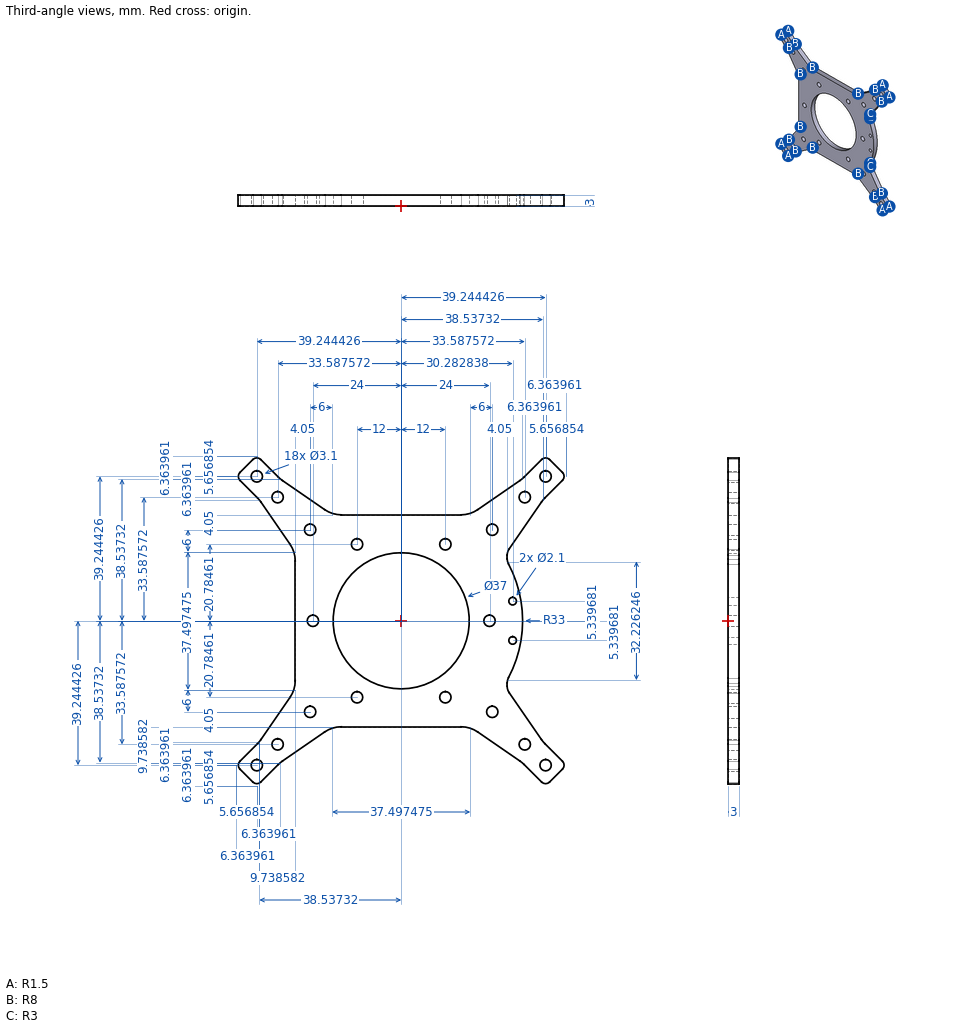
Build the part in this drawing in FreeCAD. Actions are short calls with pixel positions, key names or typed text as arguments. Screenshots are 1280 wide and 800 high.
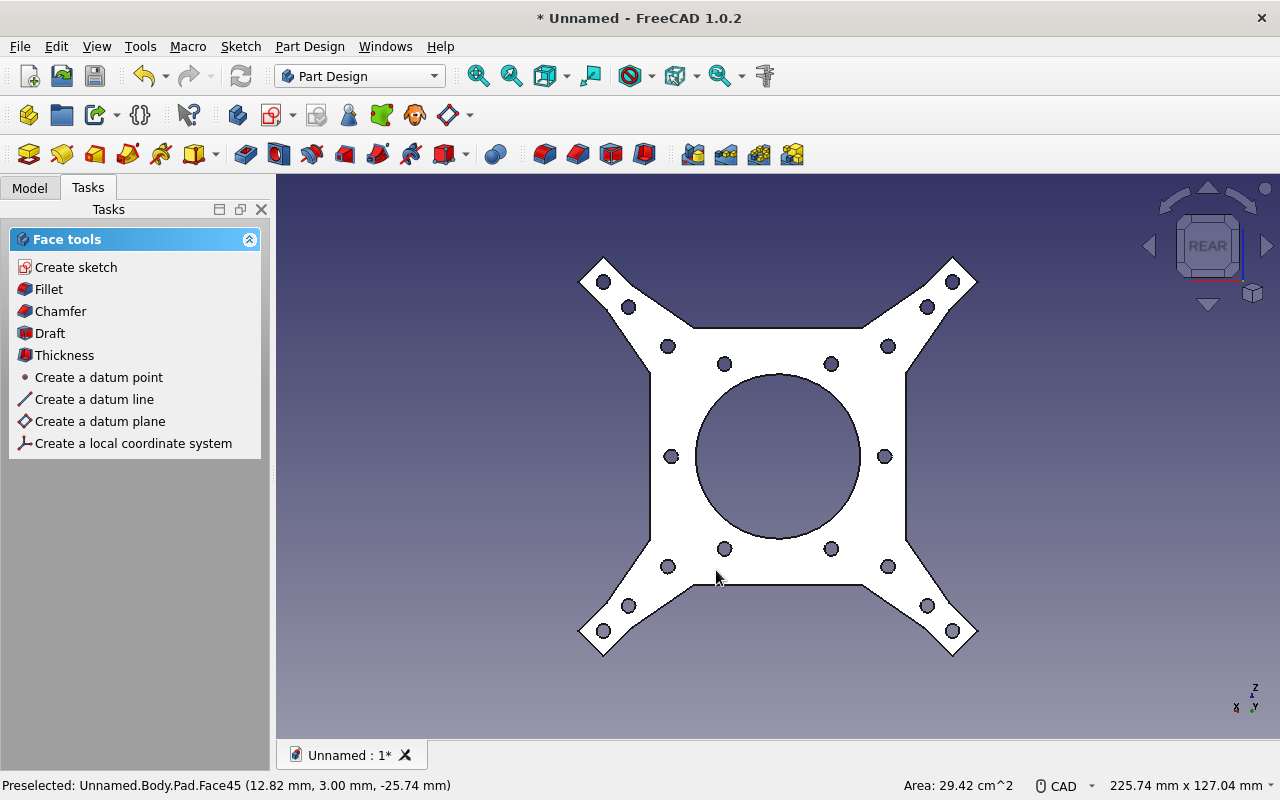
click(270, 116)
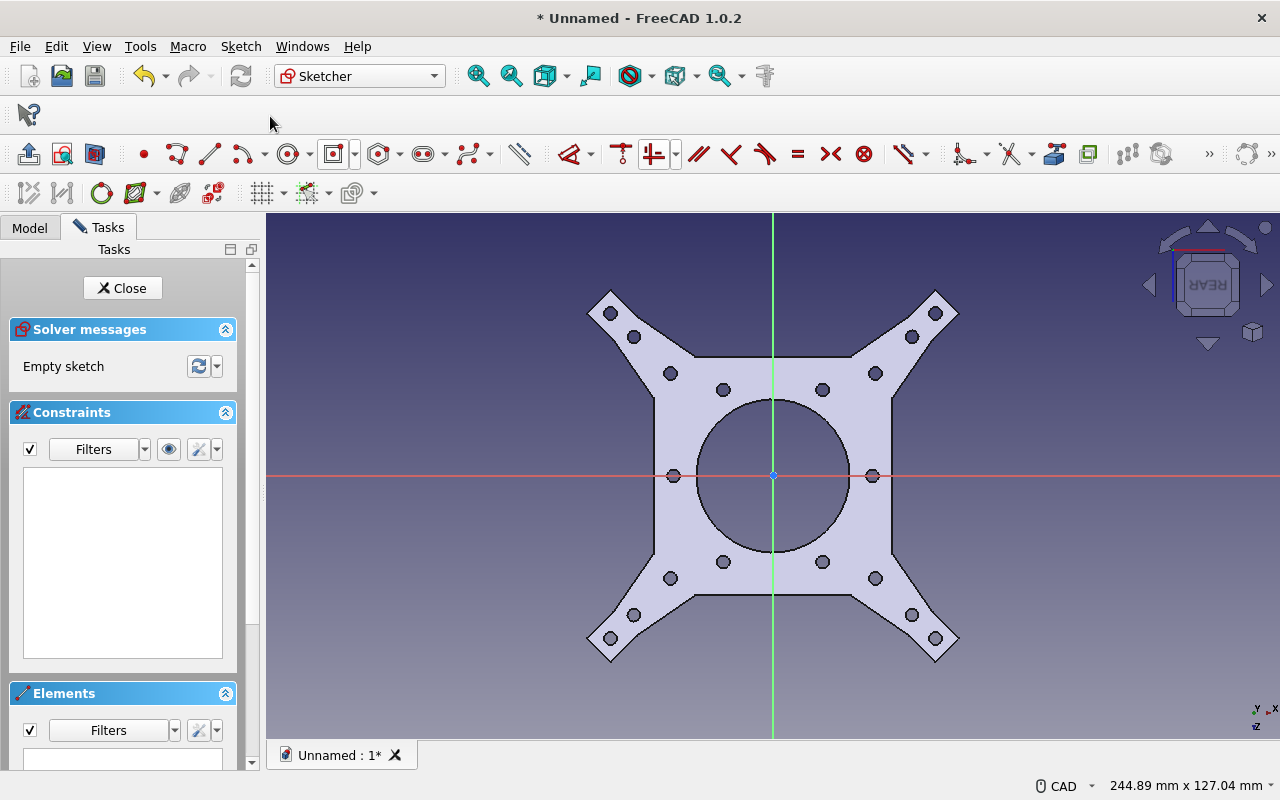
scroll(921, 476, up, 5)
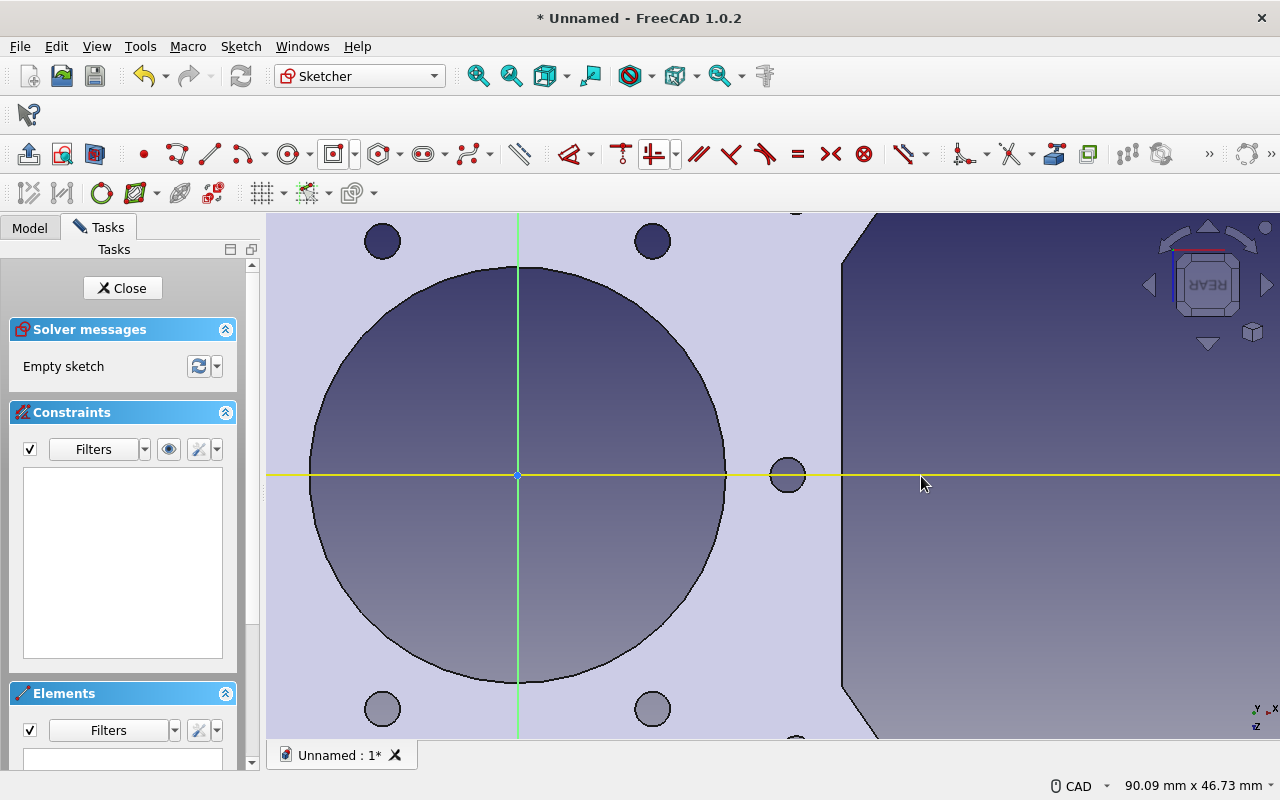
click(210, 154)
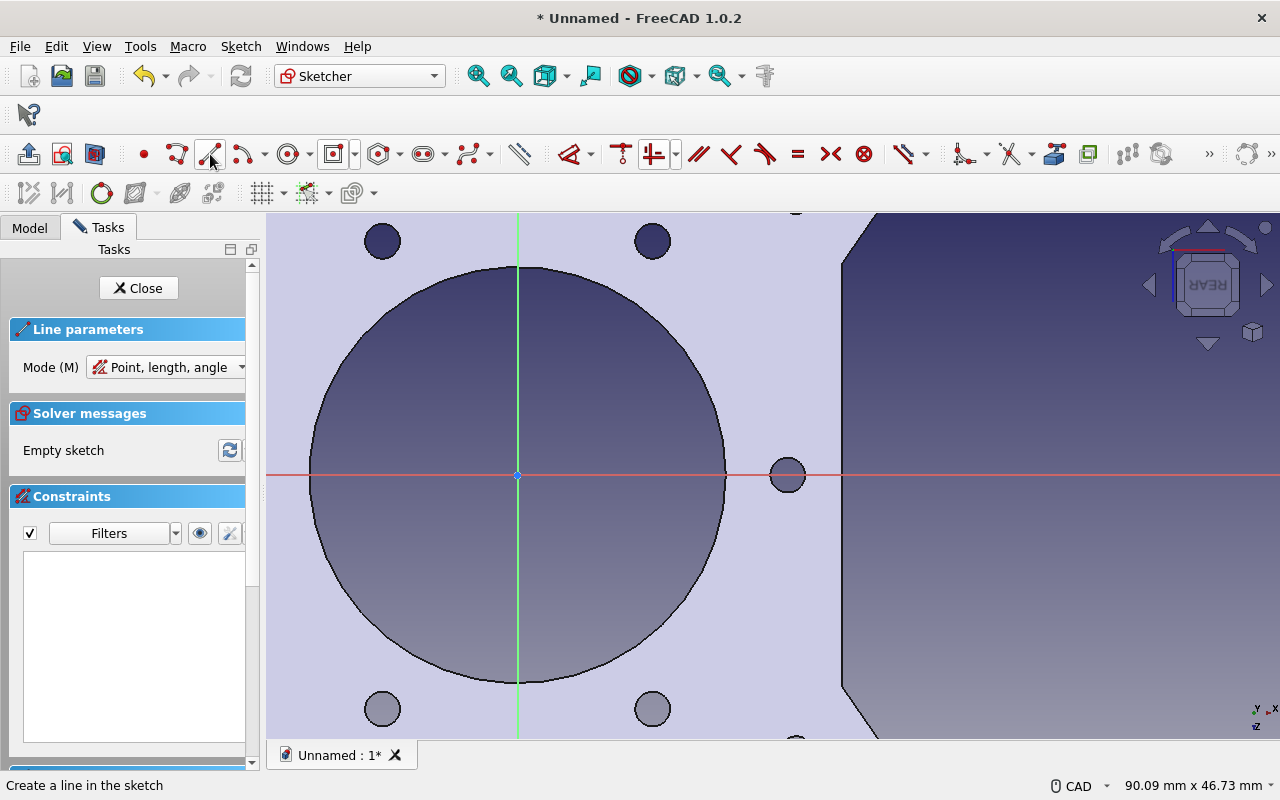
click(842, 294)
click(842, 656)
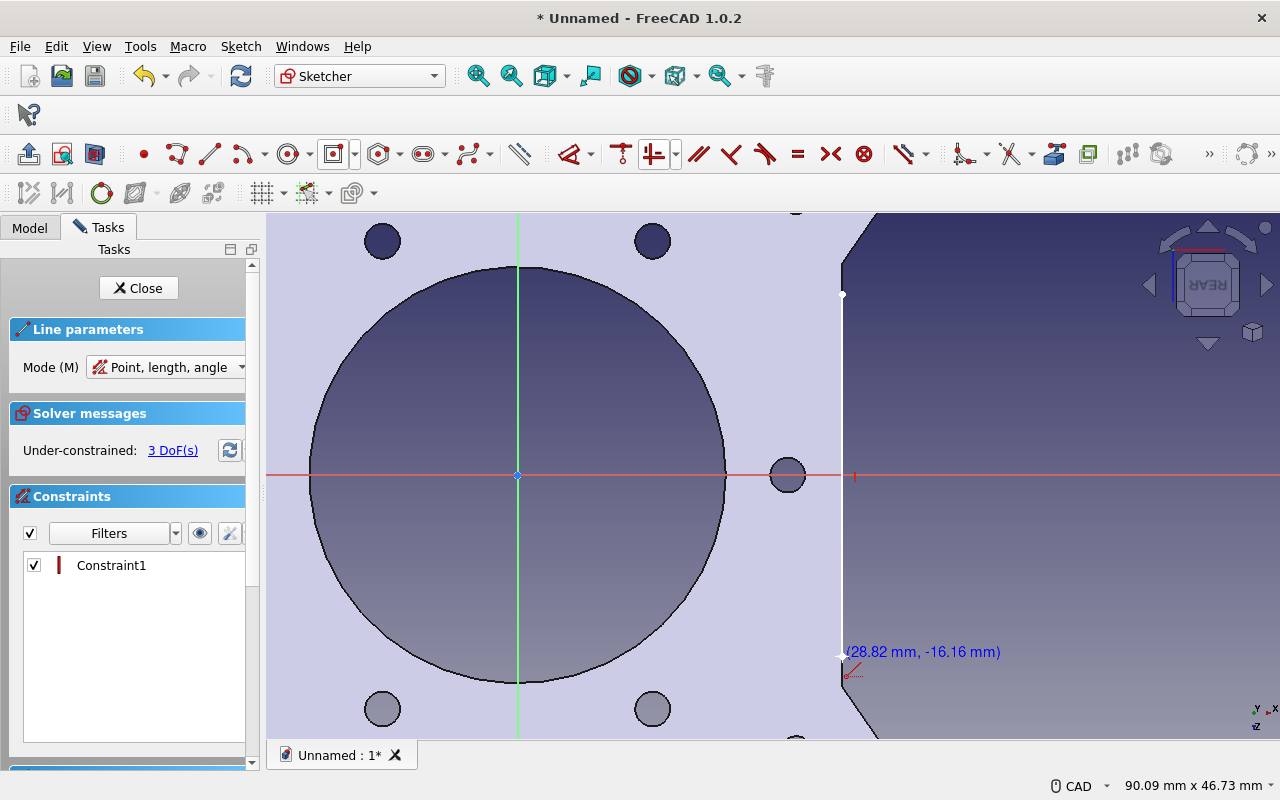
key(g)
key(3)
key(a)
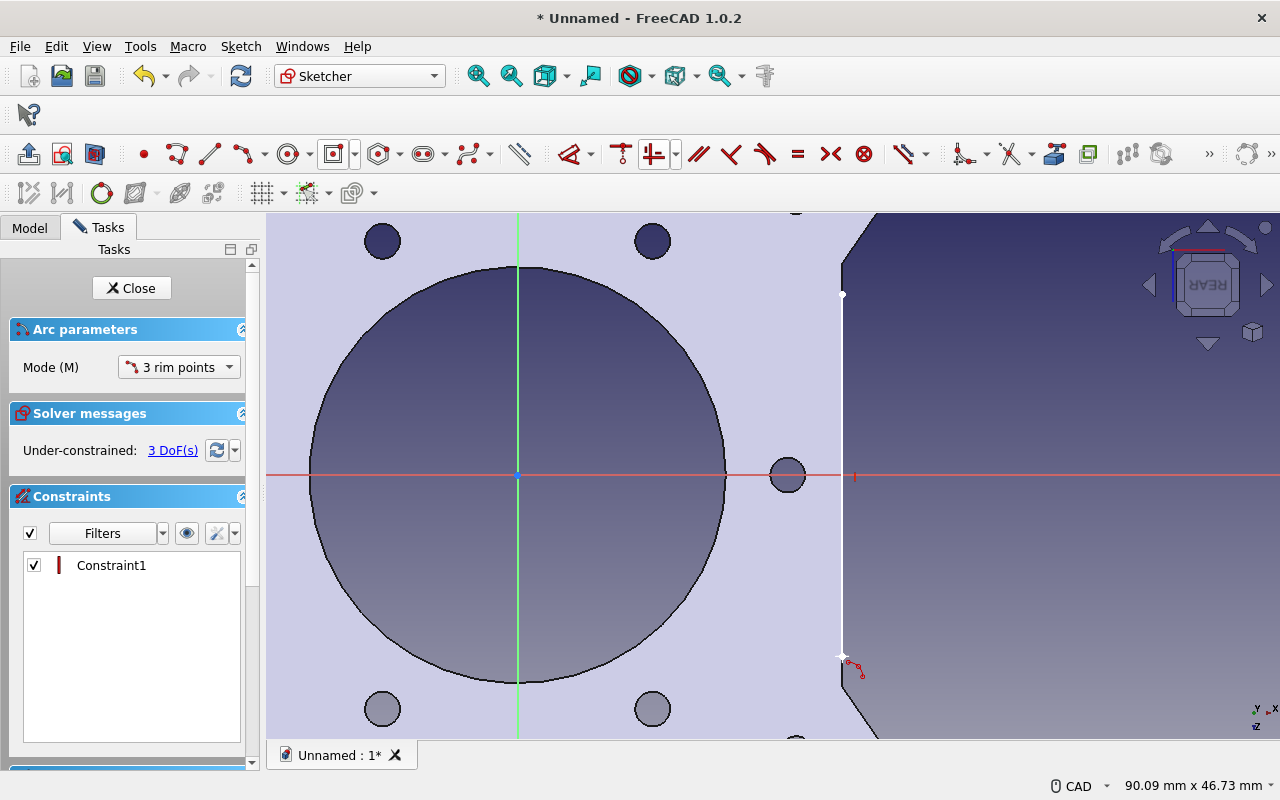
click(842, 657)
click(842, 295)
click(887, 513)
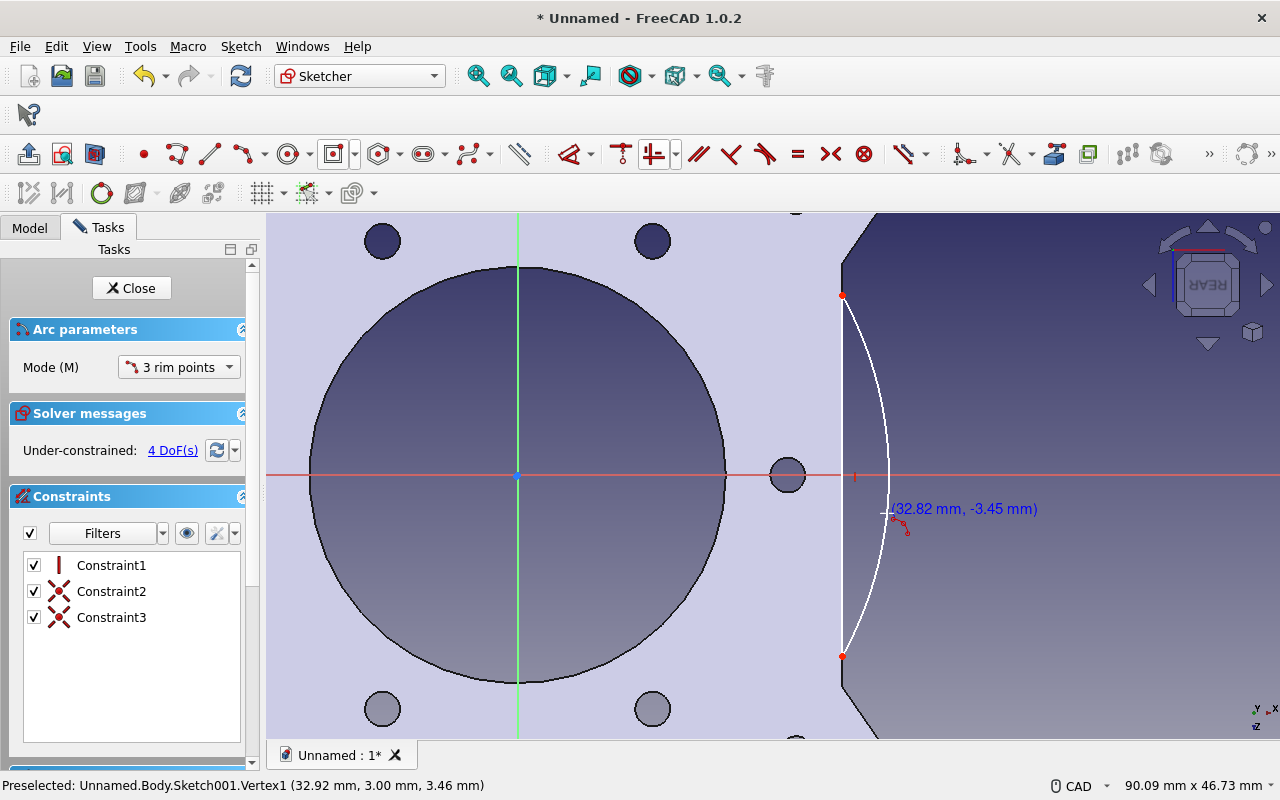
click(288, 154)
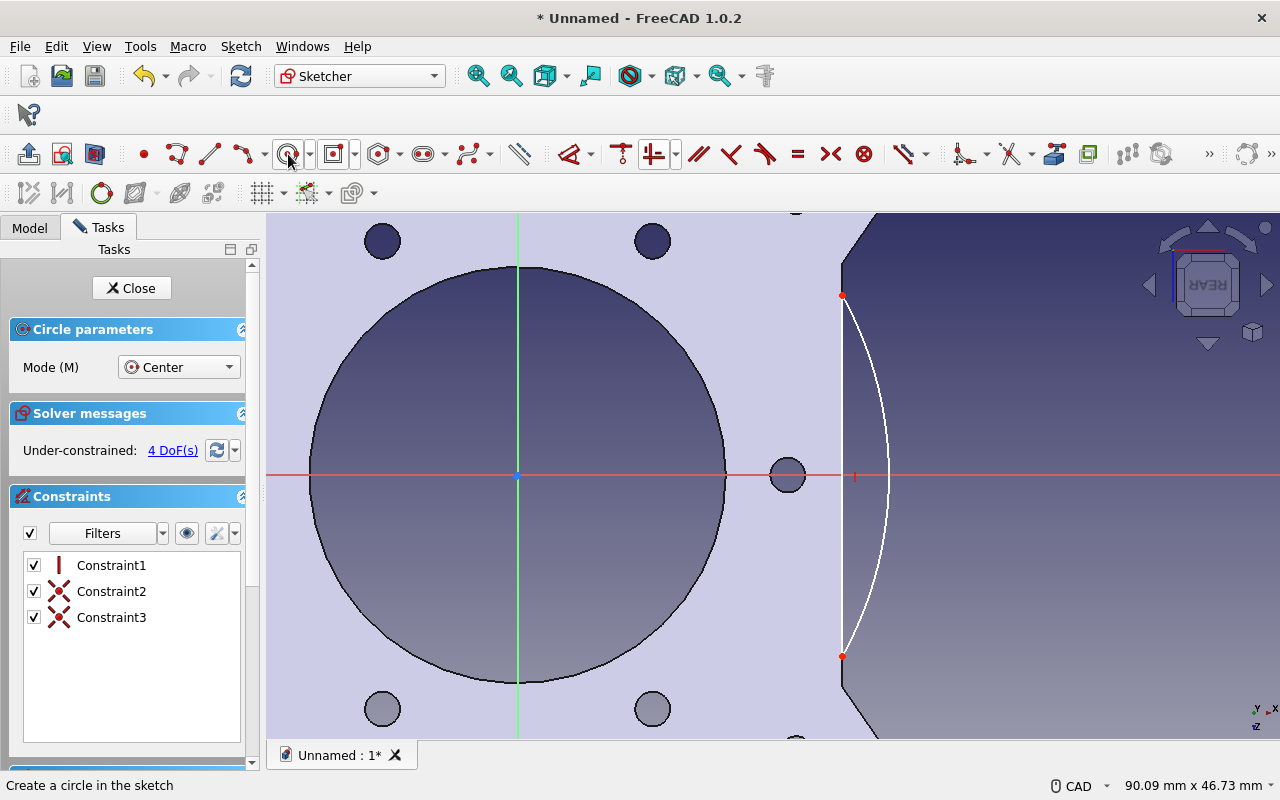
scroll(858, 535, up, 4)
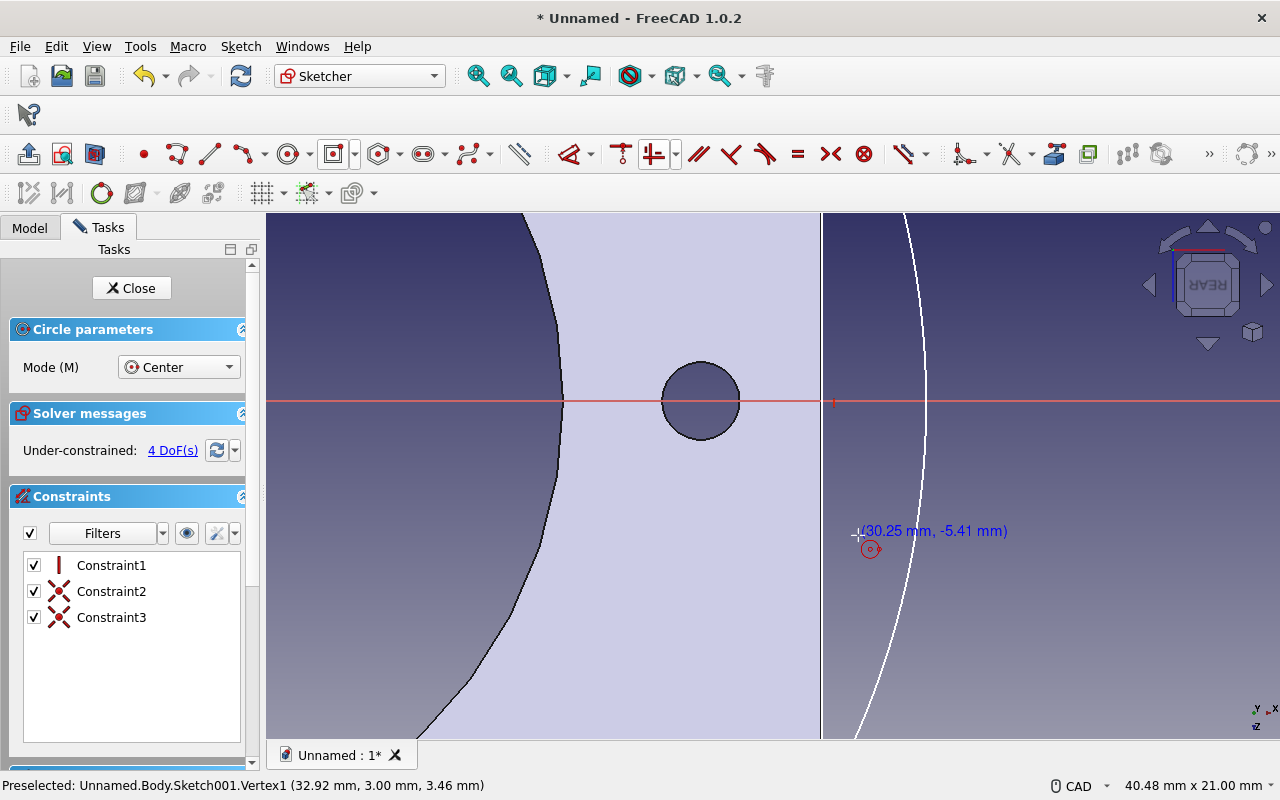
click(858, 535)
click(877, 516)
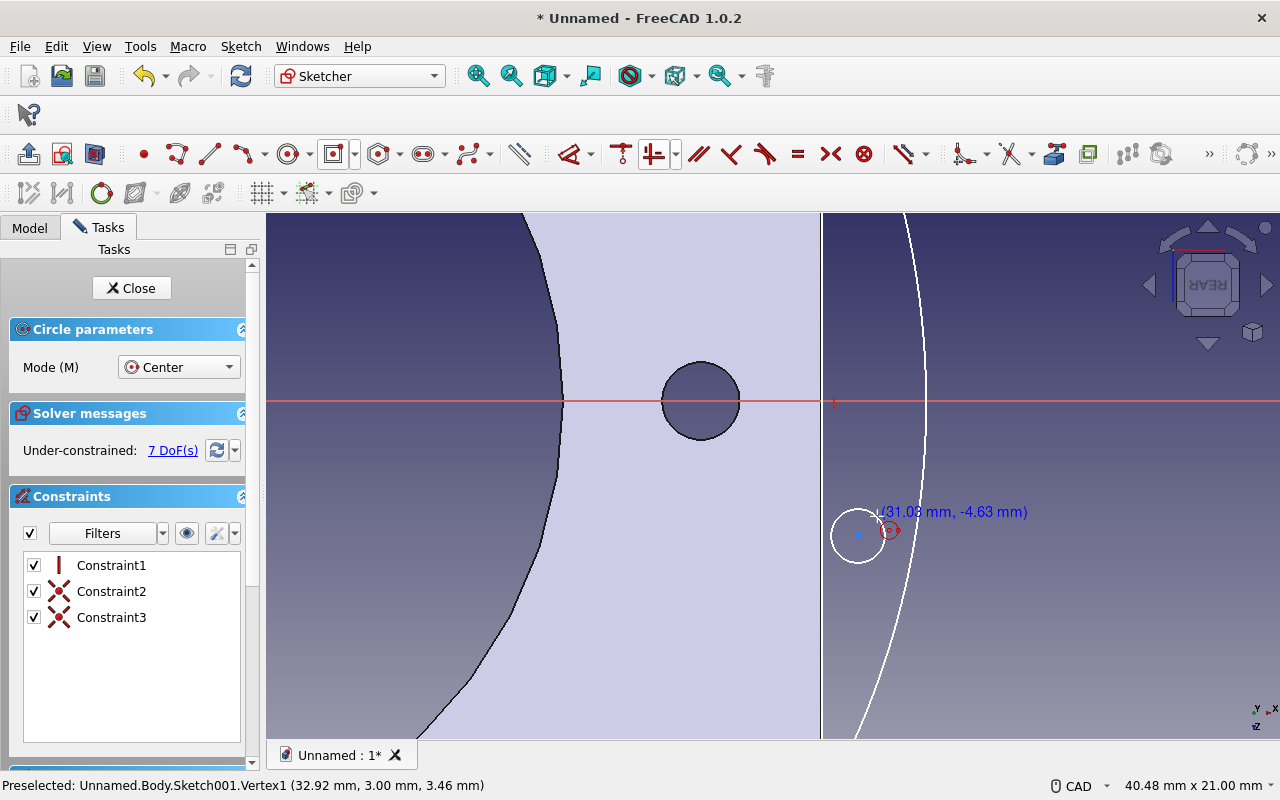
click(858, 267)
click(877, 249)
key(Escape)